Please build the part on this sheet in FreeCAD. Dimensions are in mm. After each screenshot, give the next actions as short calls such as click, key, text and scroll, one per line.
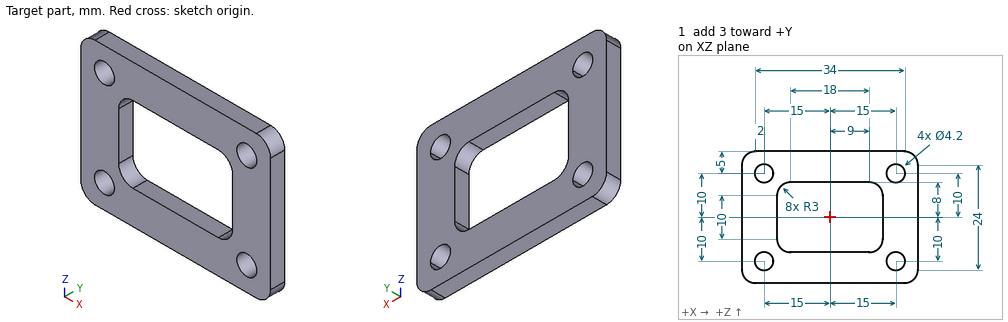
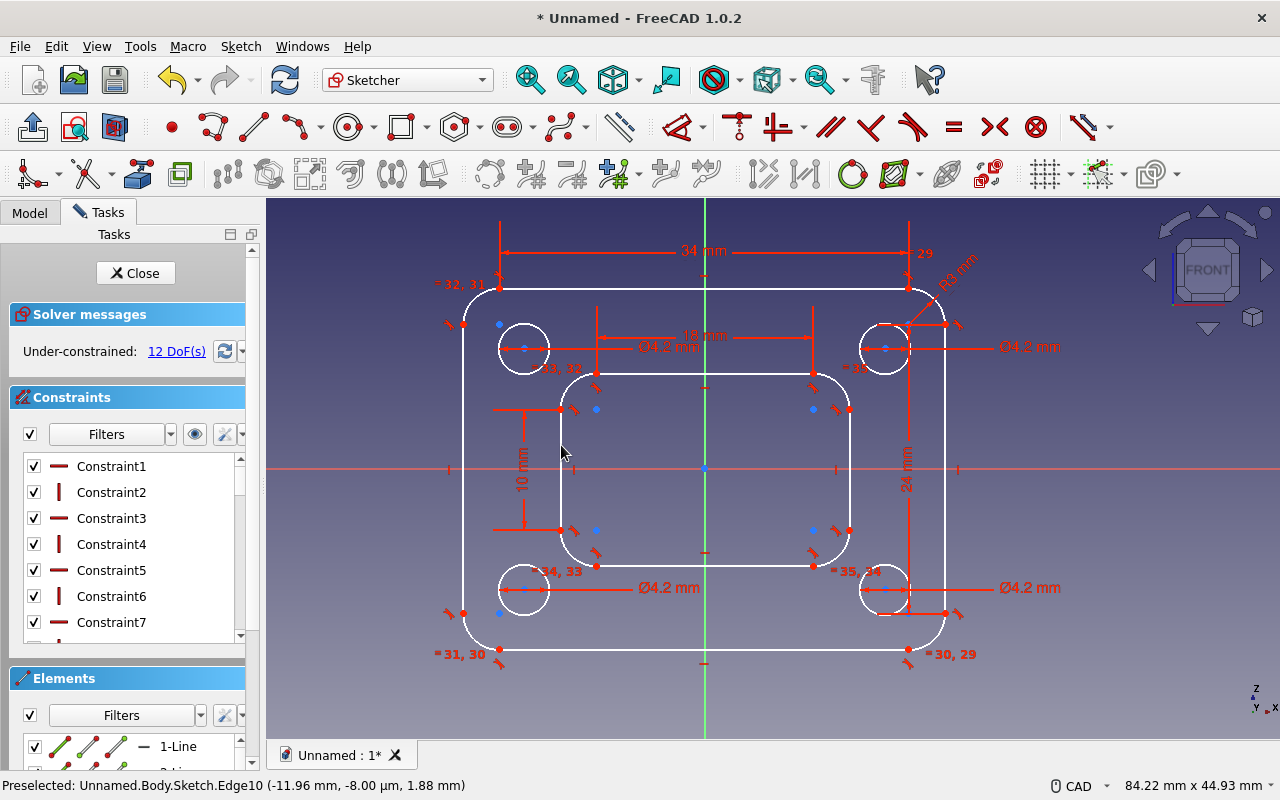
click(813, 374)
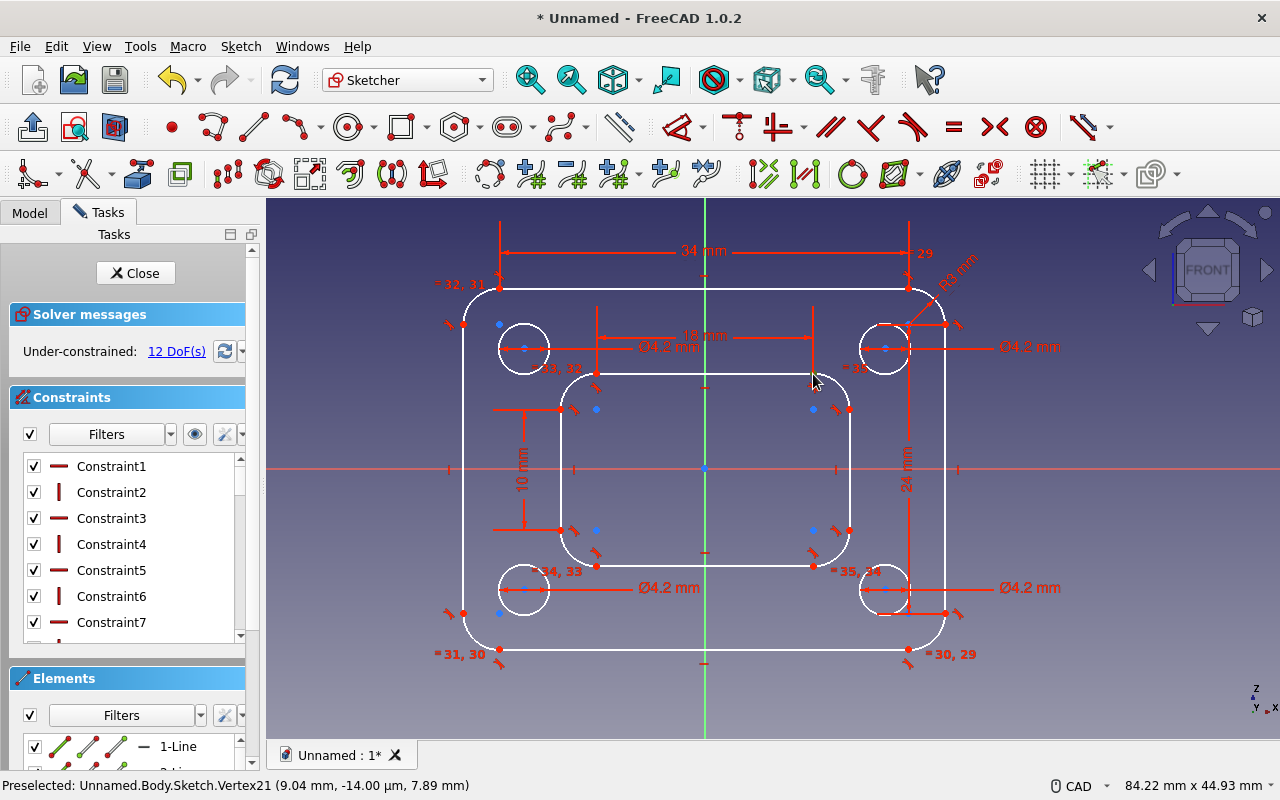
key(l)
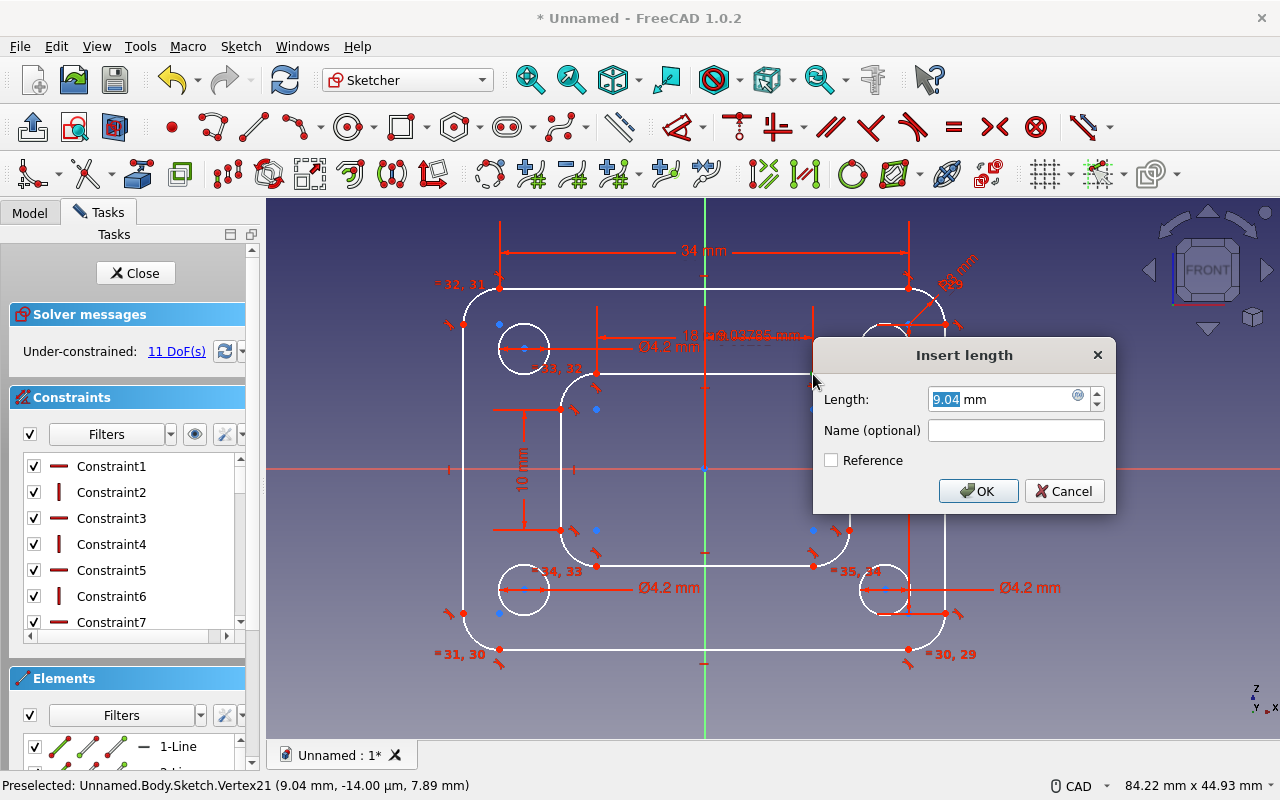
text(9)
key(Return)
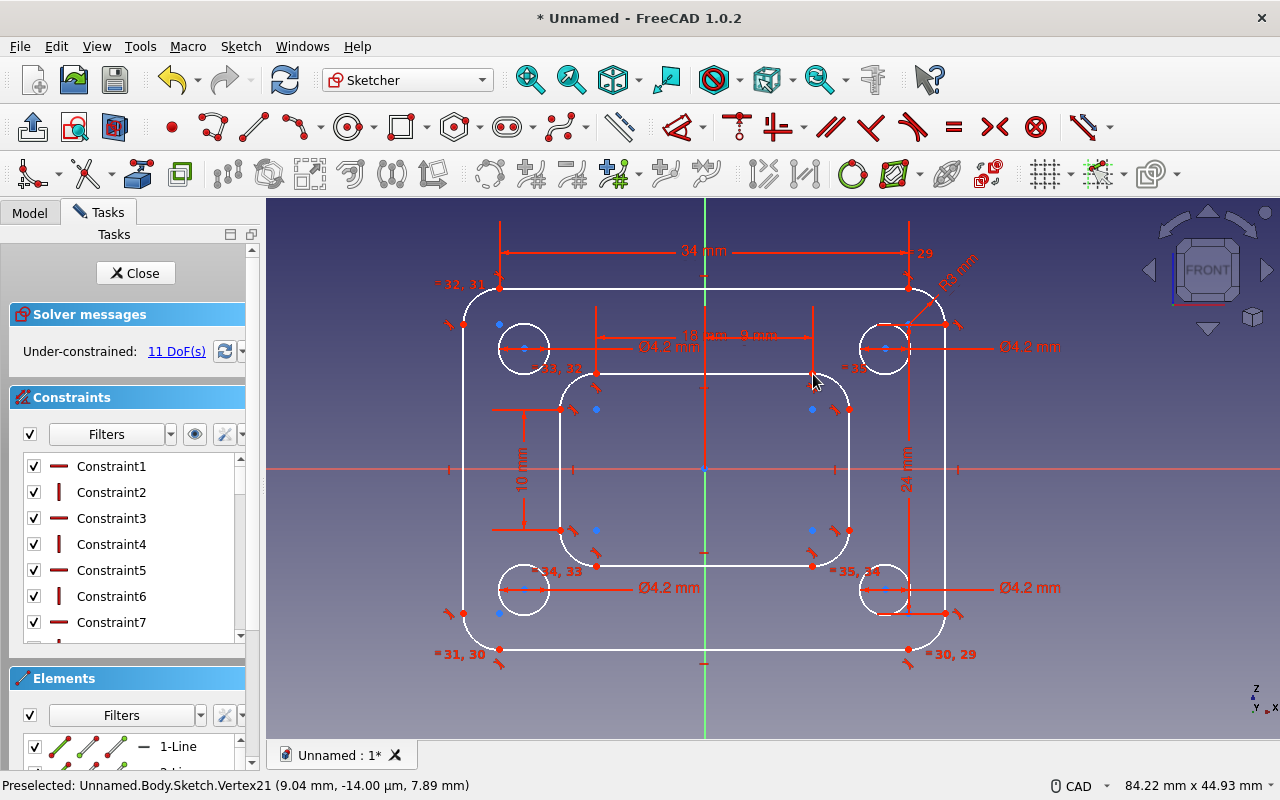
click(813, 374)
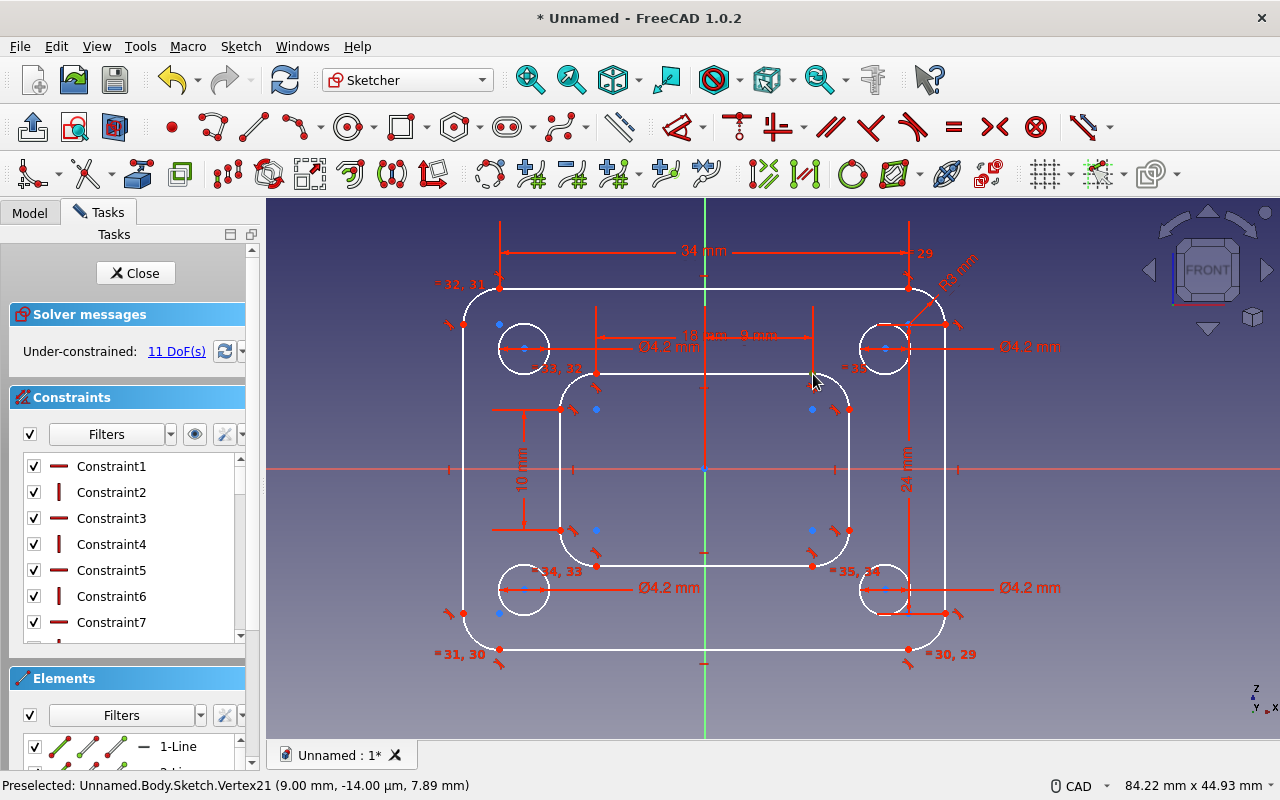
key(i)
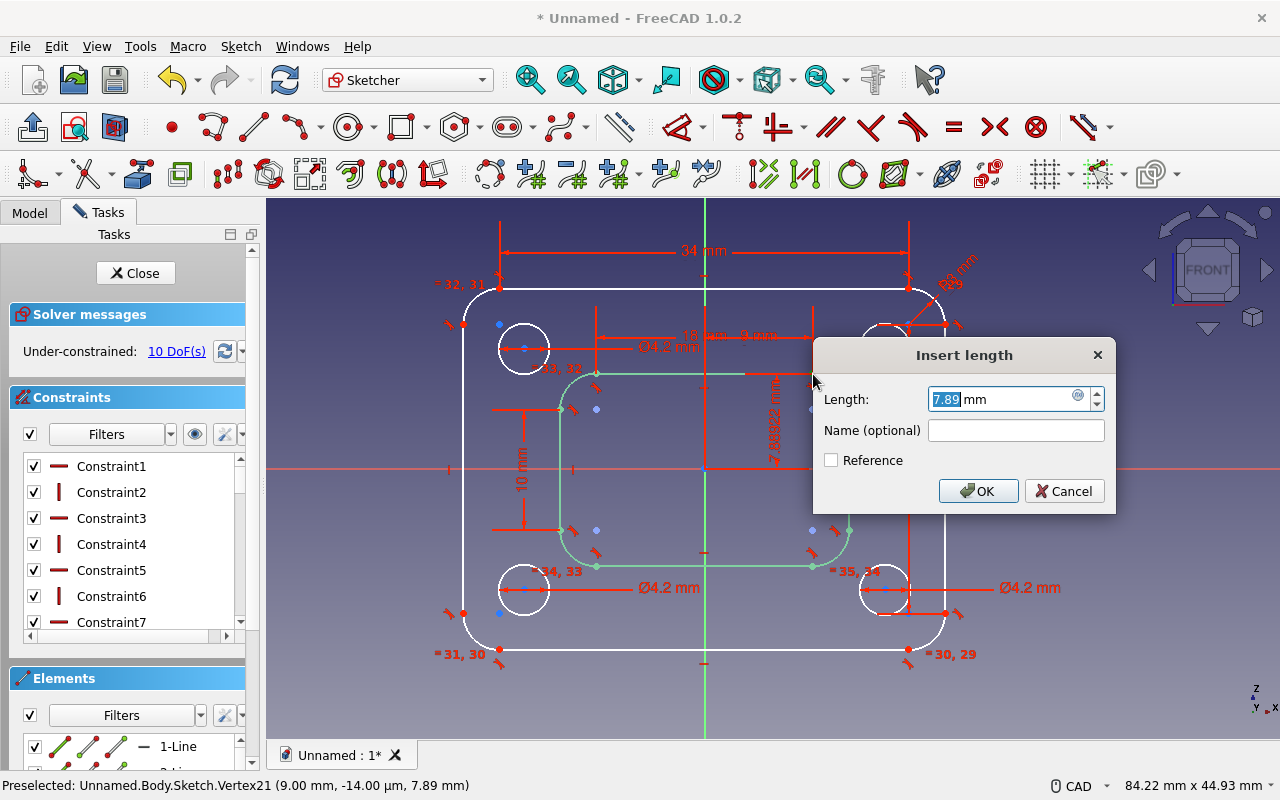
text(8)
key(Return)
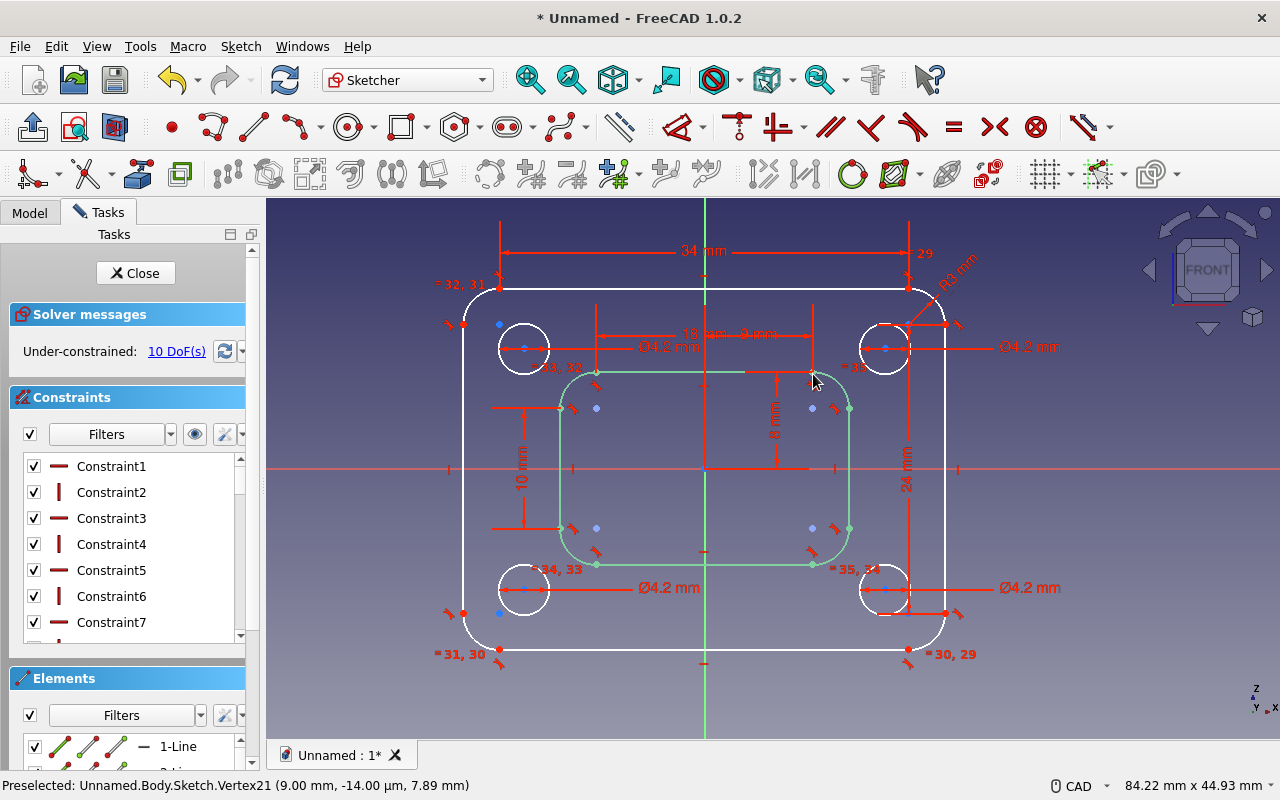
click(524, 349)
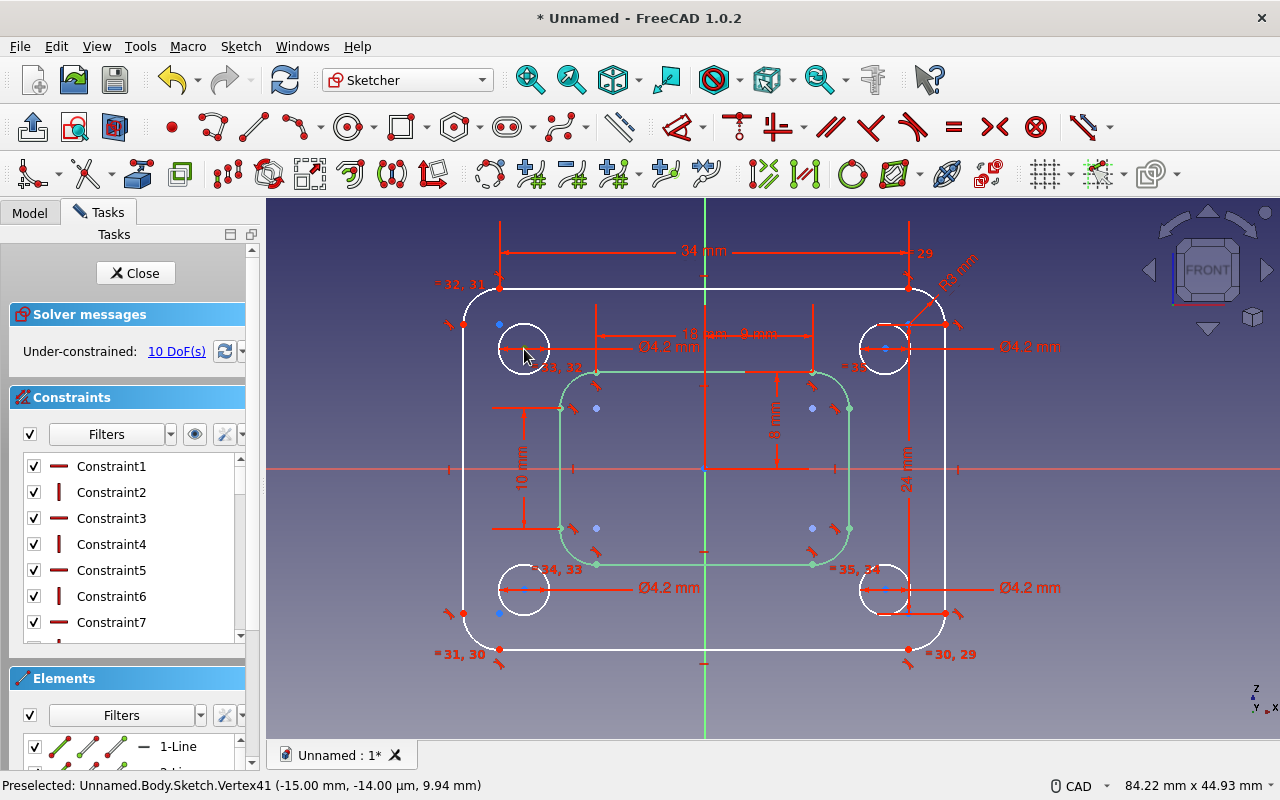
key(l)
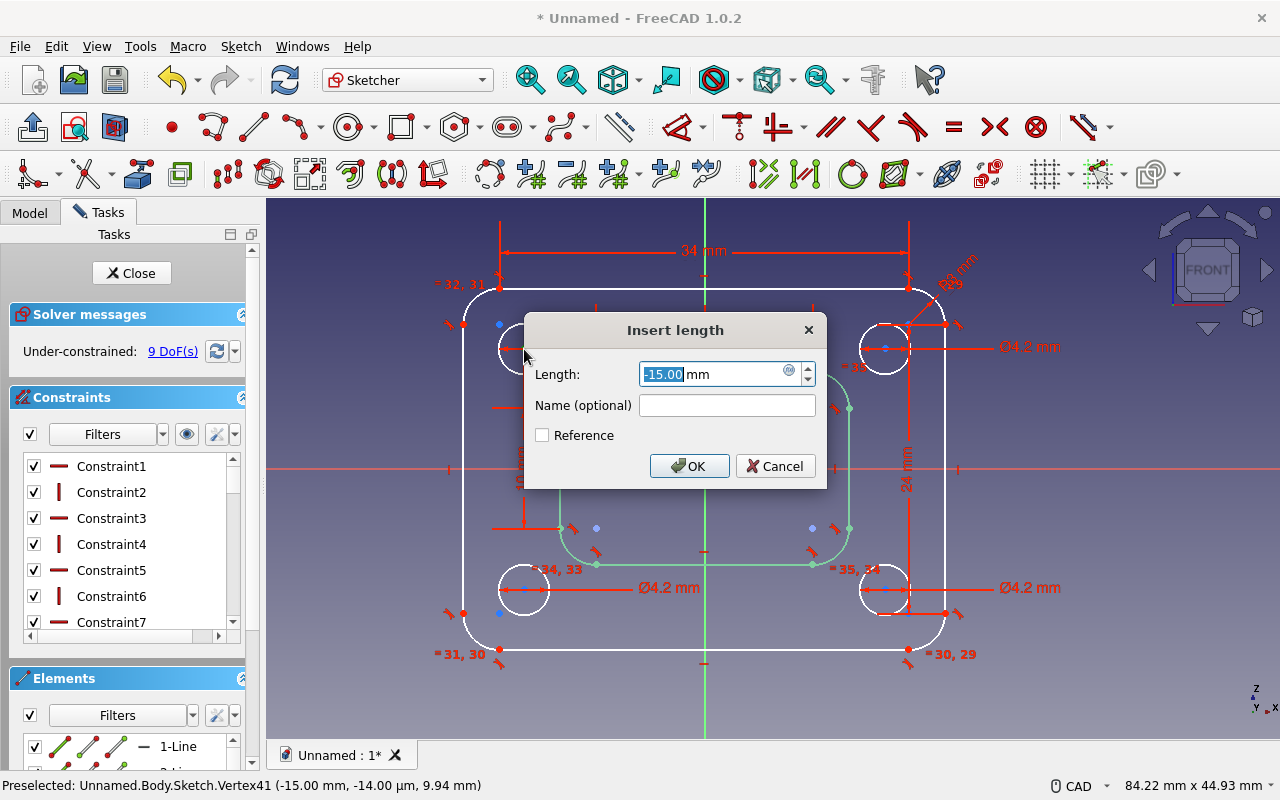
text(-15)
key(Return)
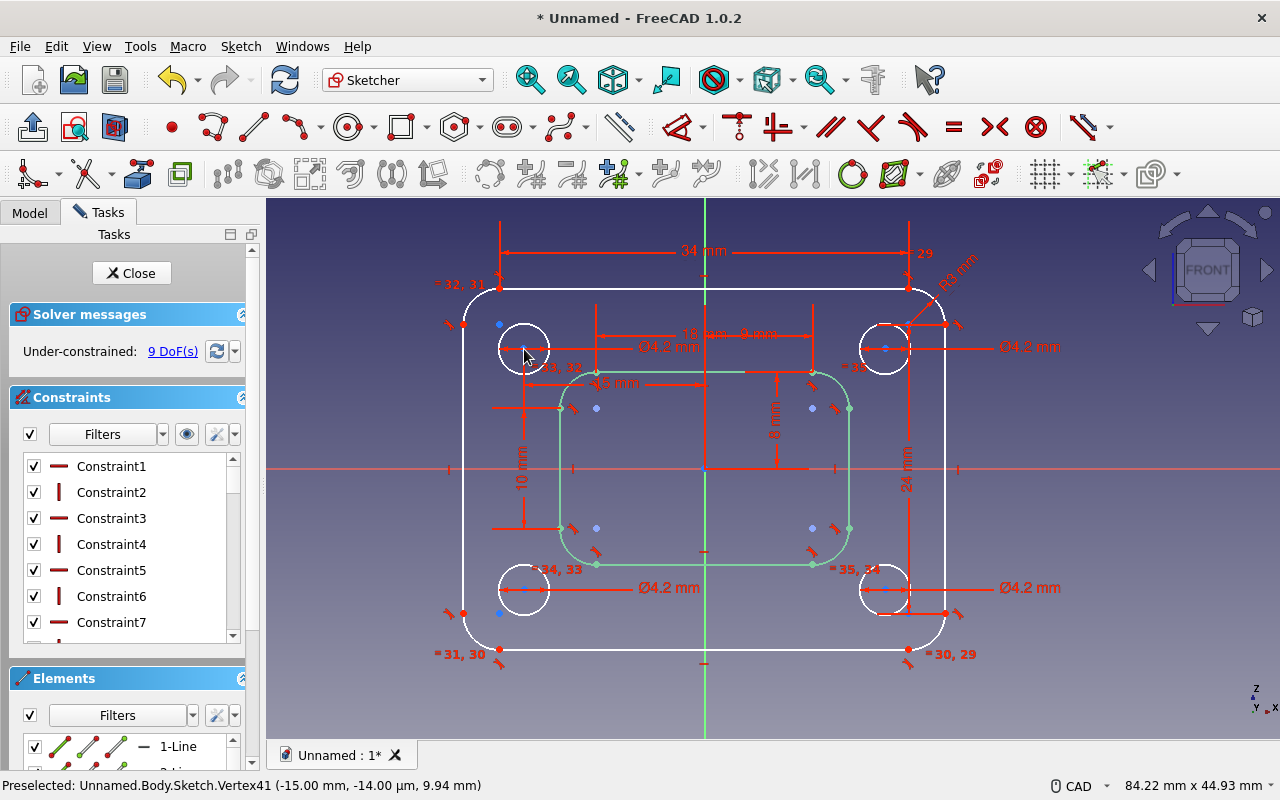
click(524, 349)